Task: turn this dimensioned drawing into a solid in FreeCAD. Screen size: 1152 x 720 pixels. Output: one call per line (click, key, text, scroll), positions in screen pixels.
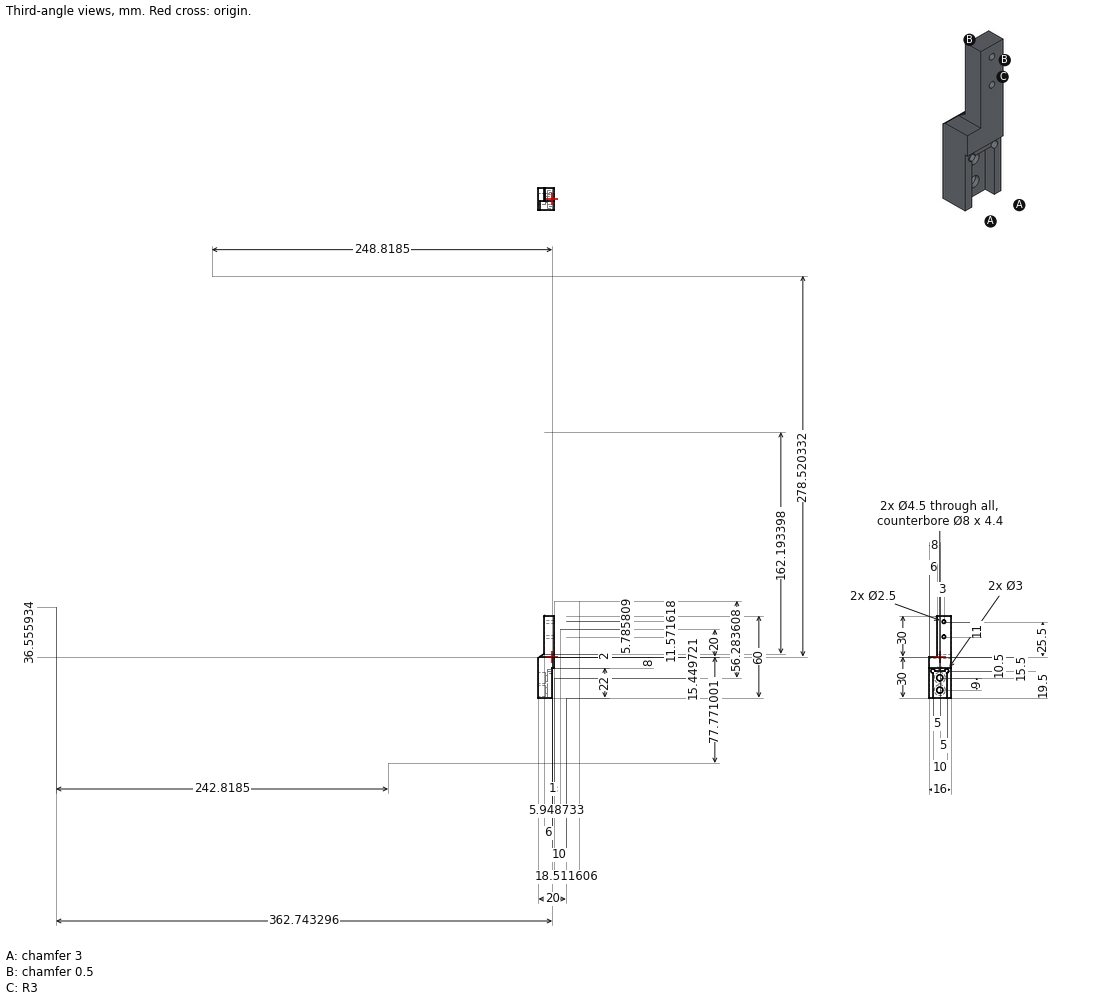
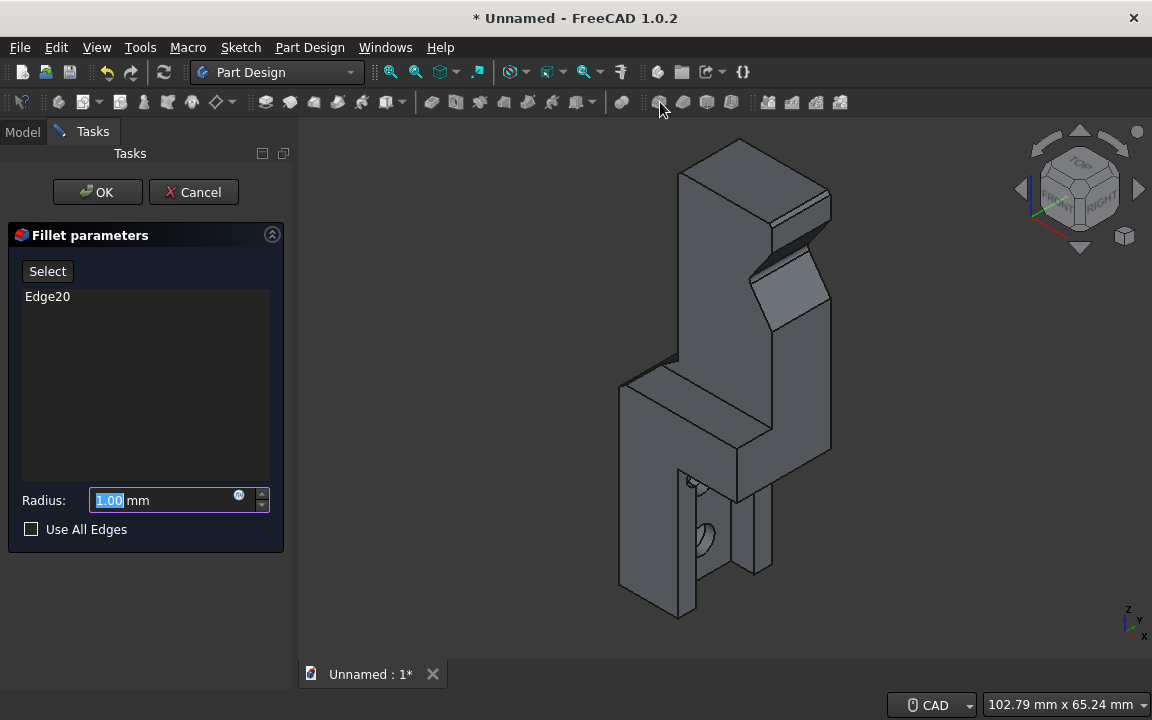
text(3)
key(Tab)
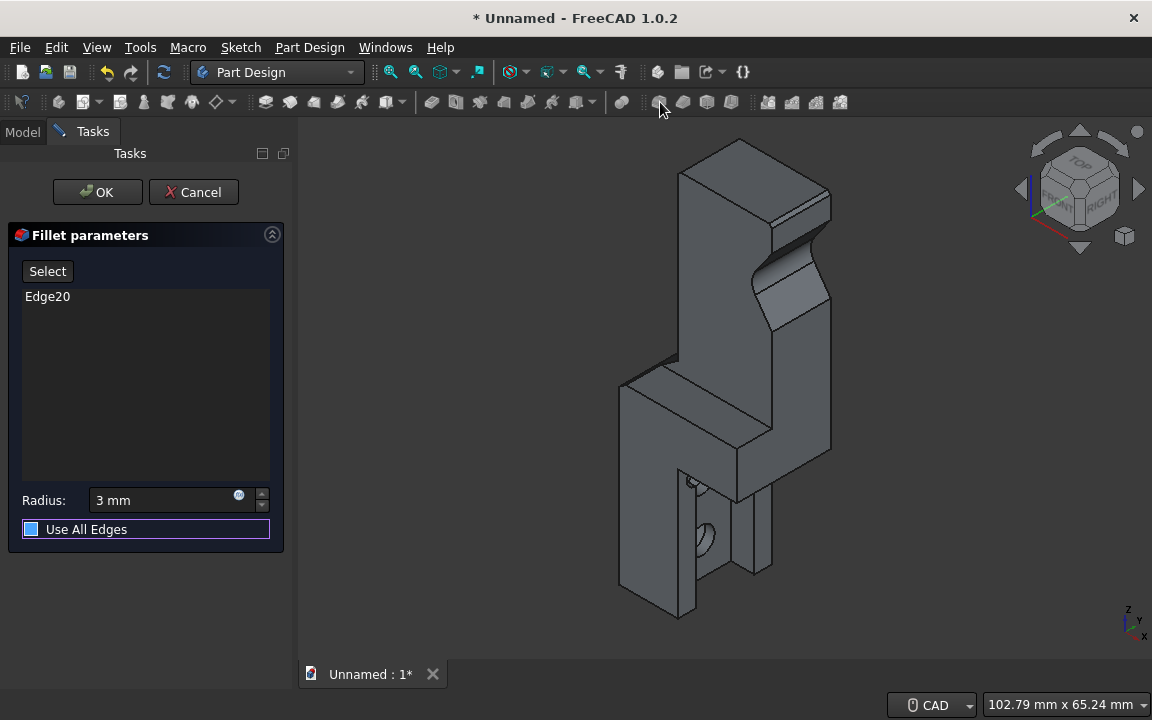
click(98, 192)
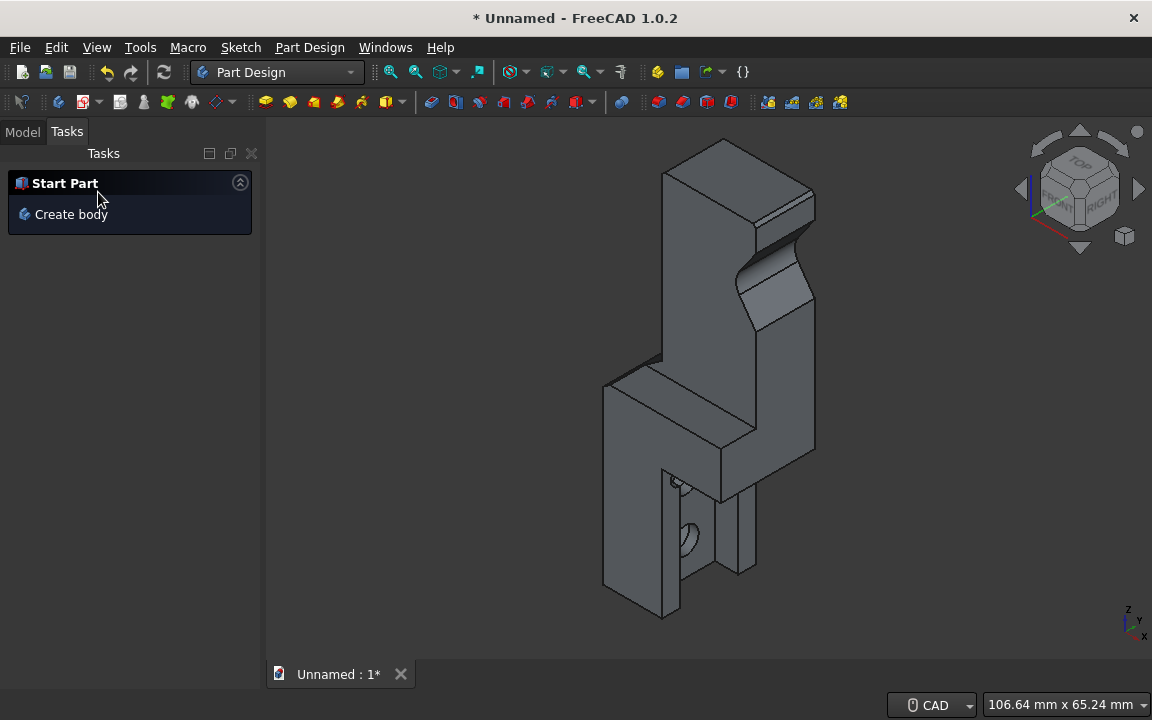
key(4)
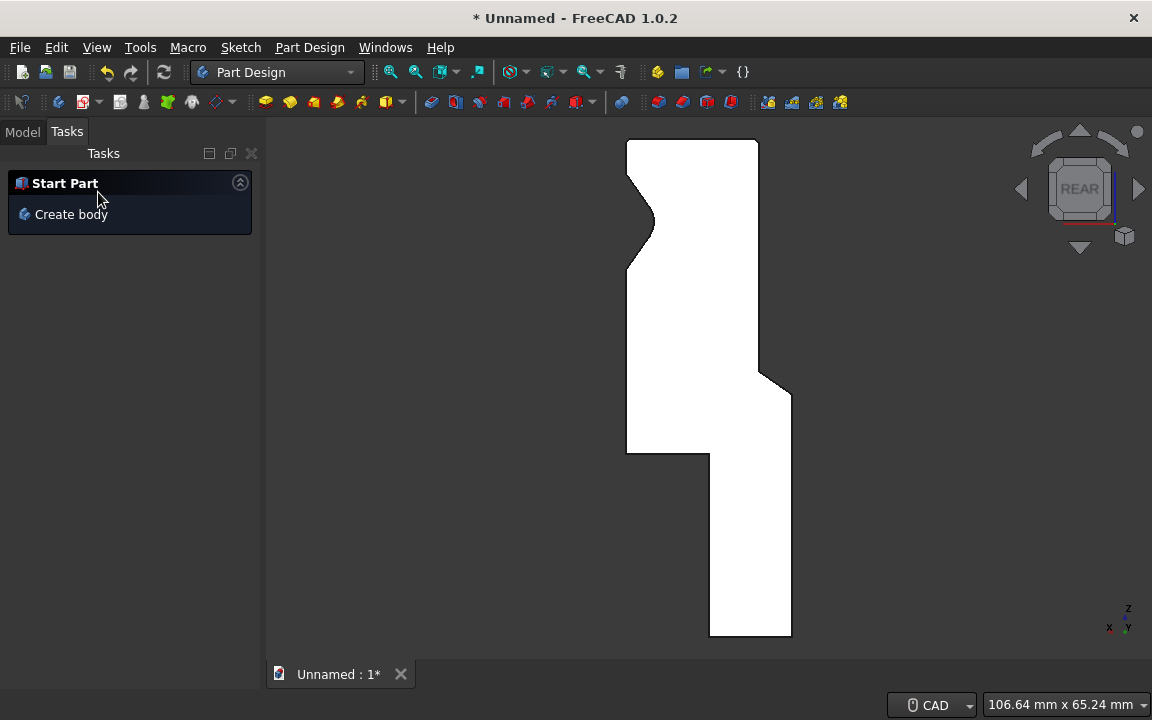
click(685, 316)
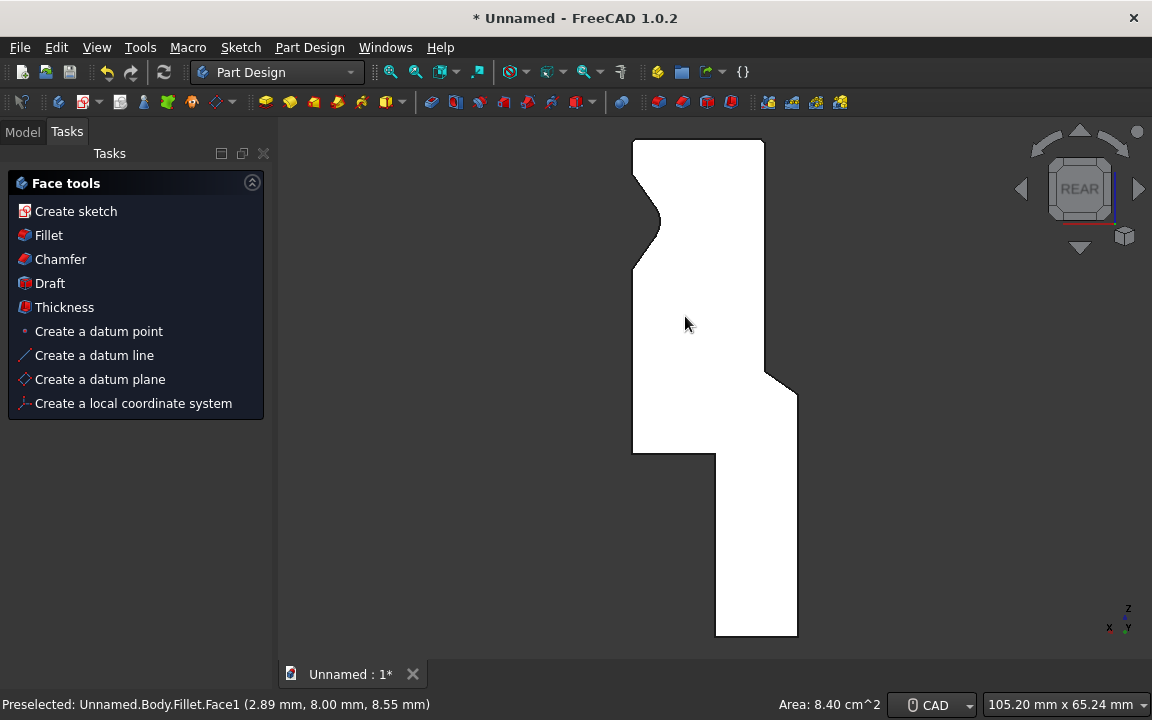
click(84, 102)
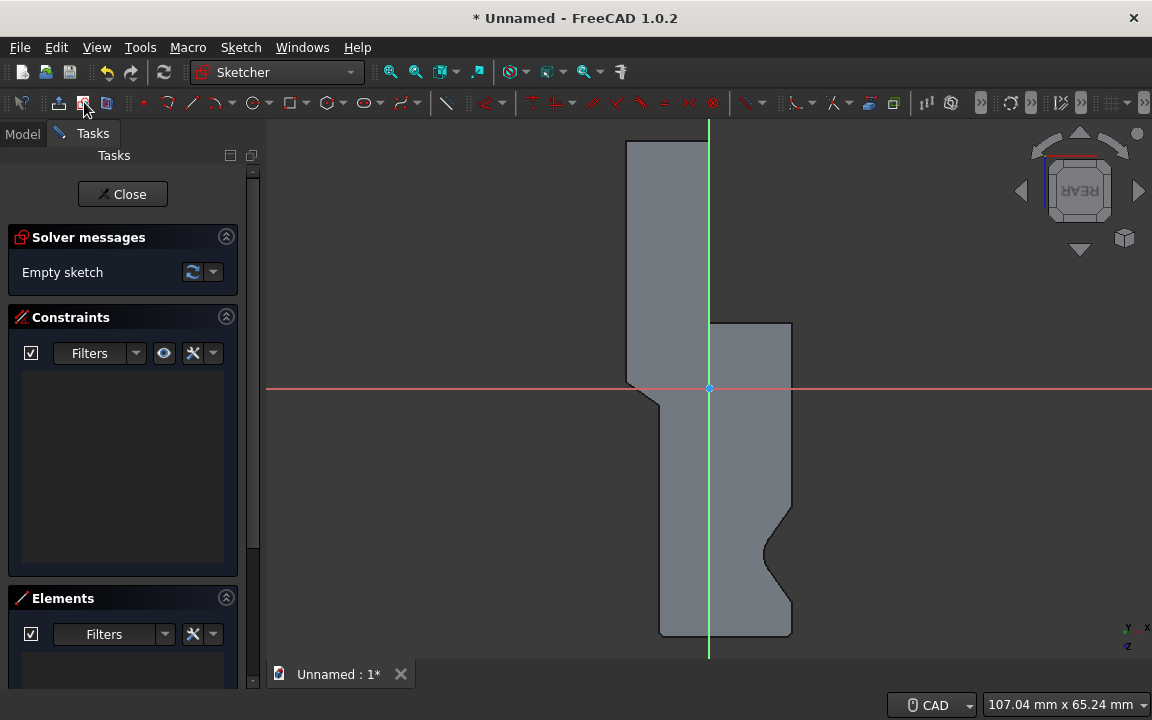
scroll(337, 175, down, 2)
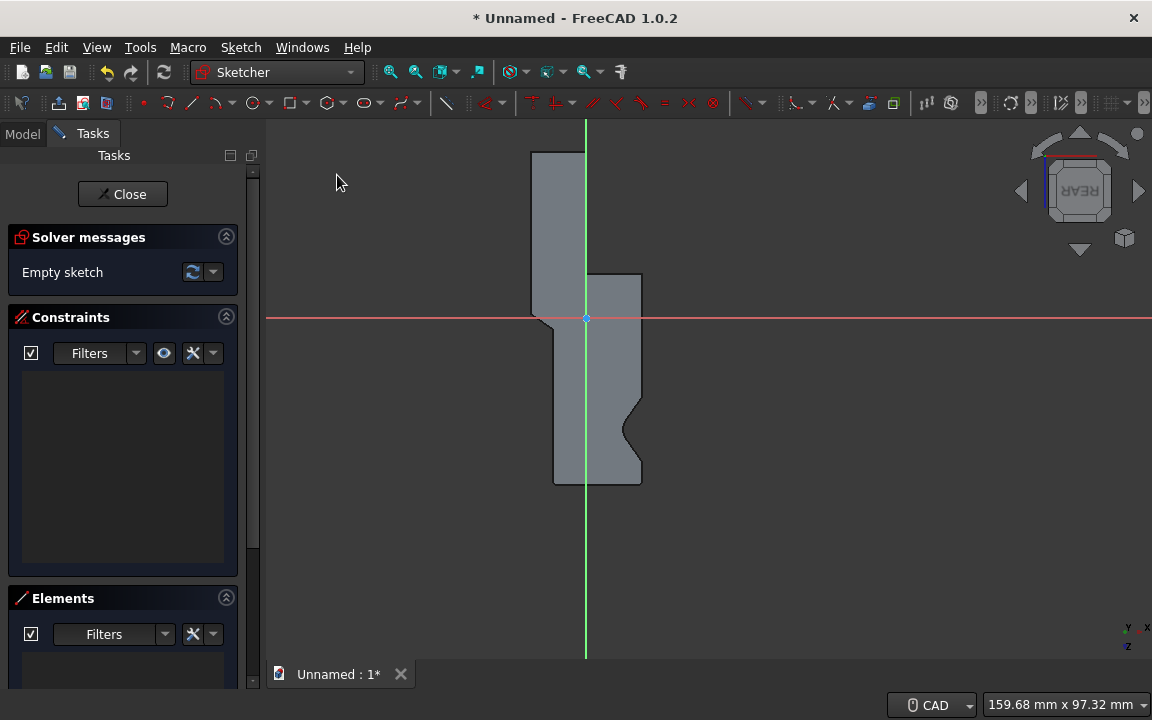
key(g)
key(r)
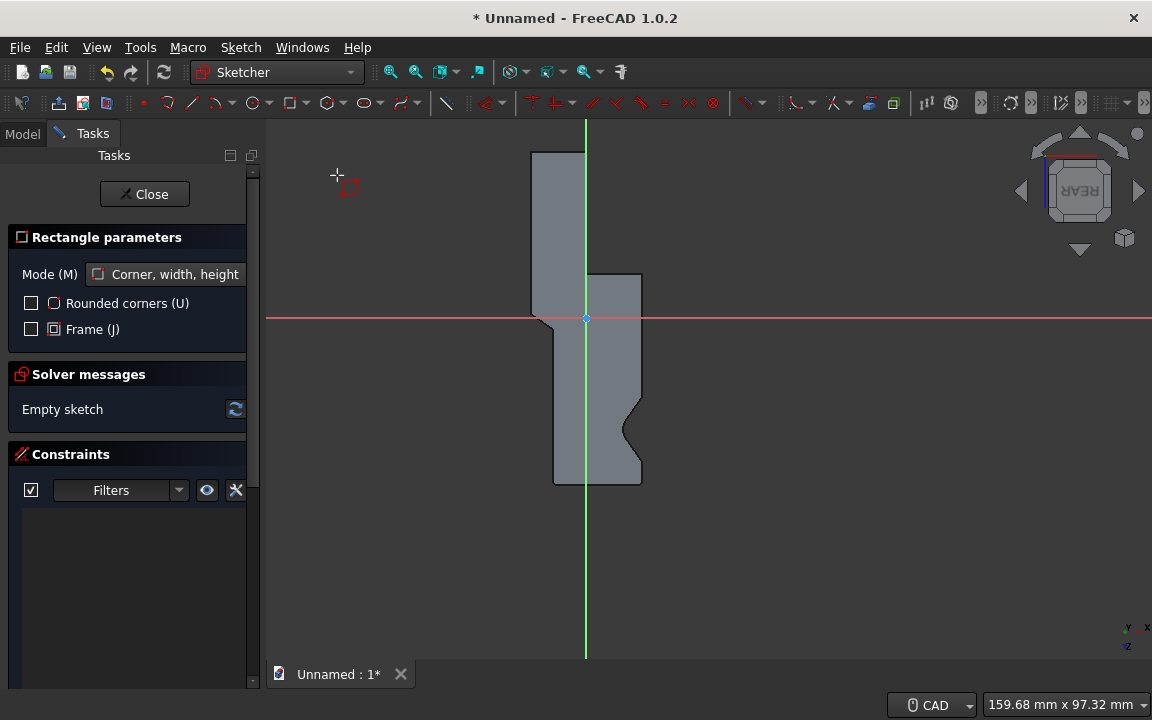
scroll(592, 233, up, 6)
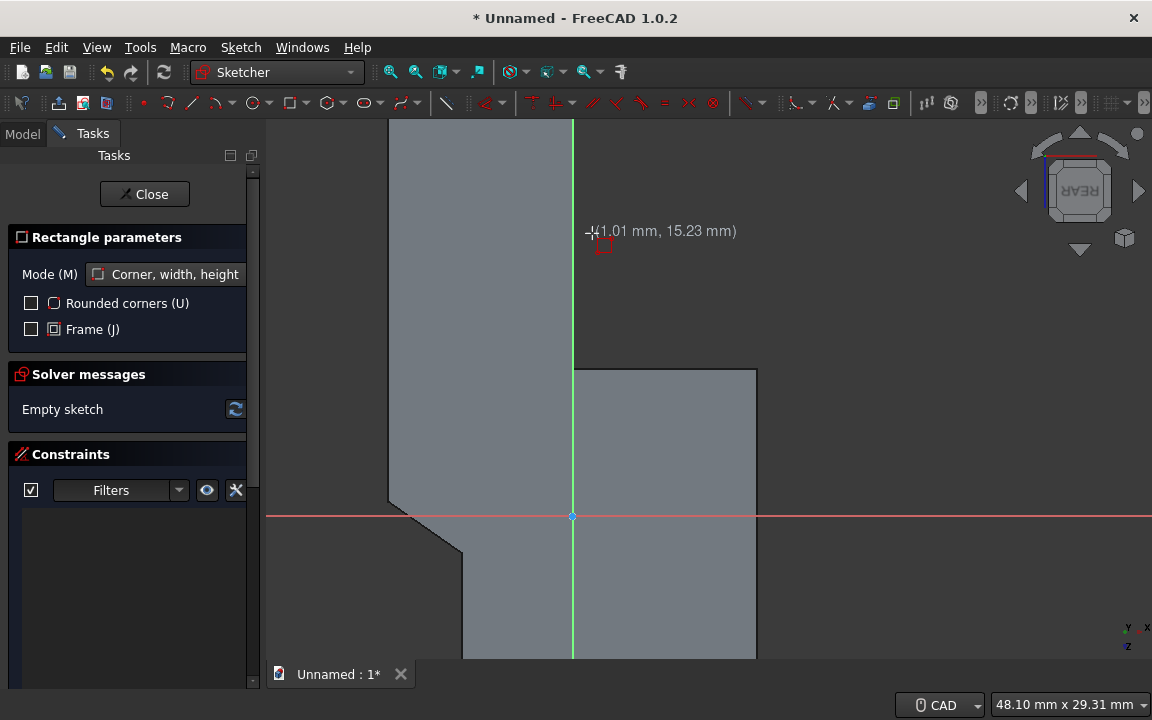
click(591, 232)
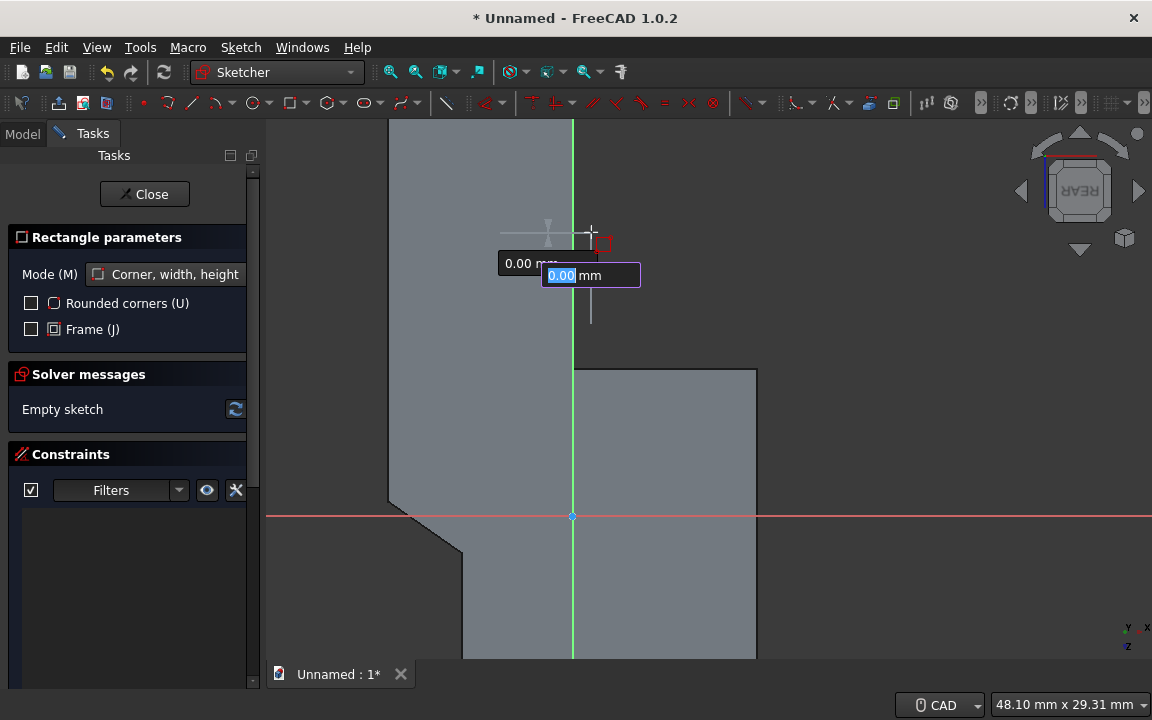
scroll(592, 233, down, 6)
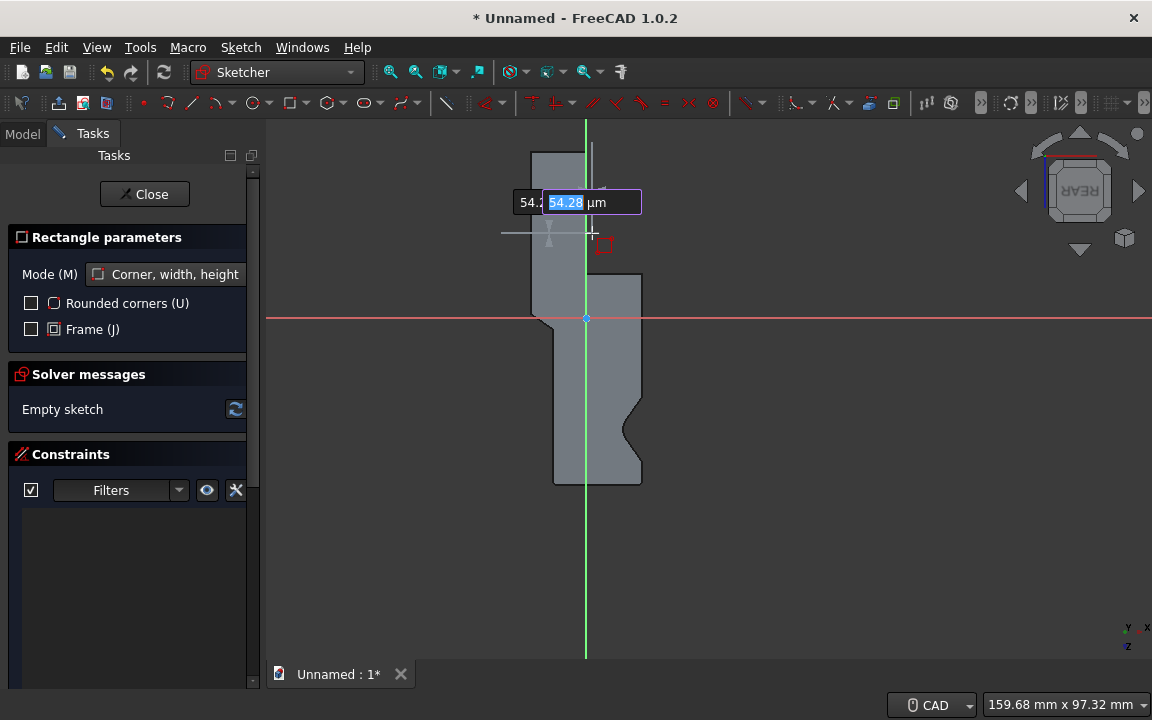
click(695, 545)
key(Escape)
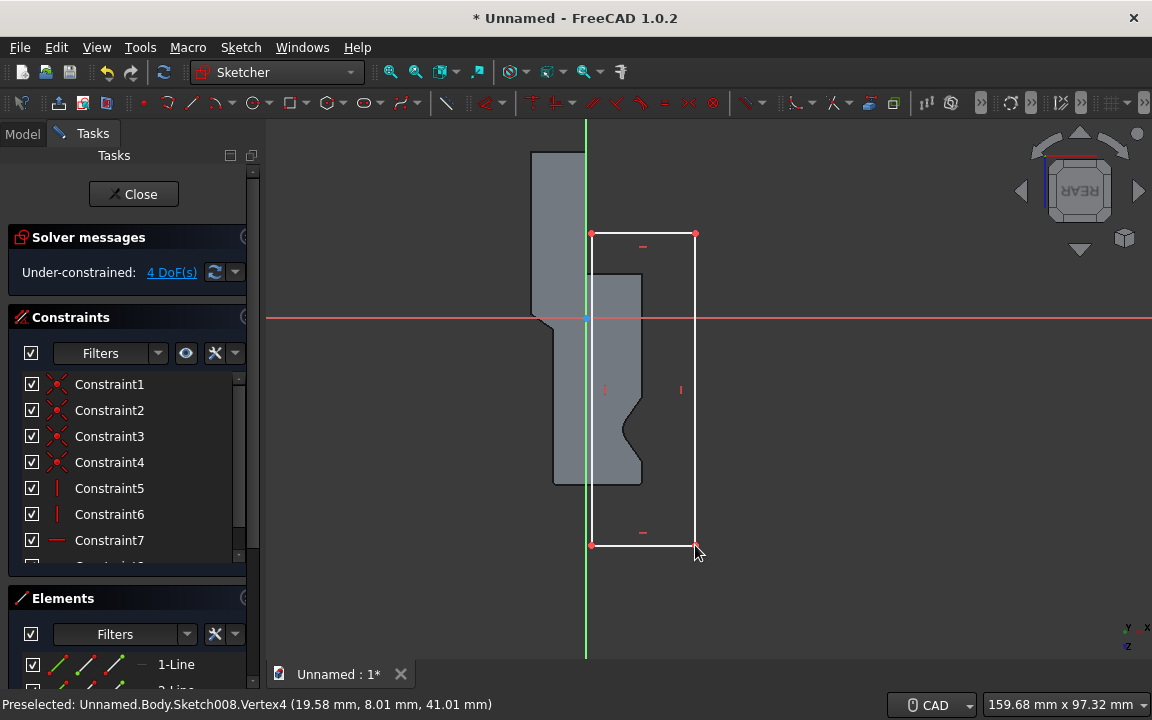
key(d)